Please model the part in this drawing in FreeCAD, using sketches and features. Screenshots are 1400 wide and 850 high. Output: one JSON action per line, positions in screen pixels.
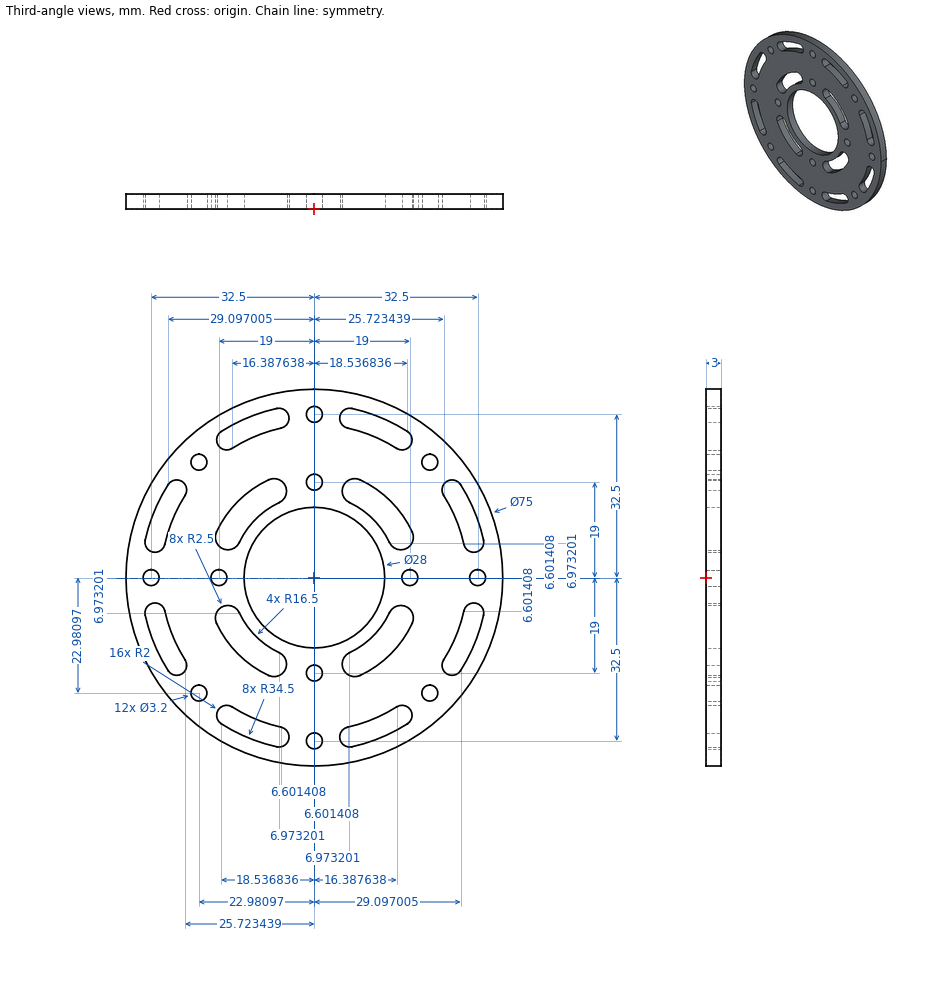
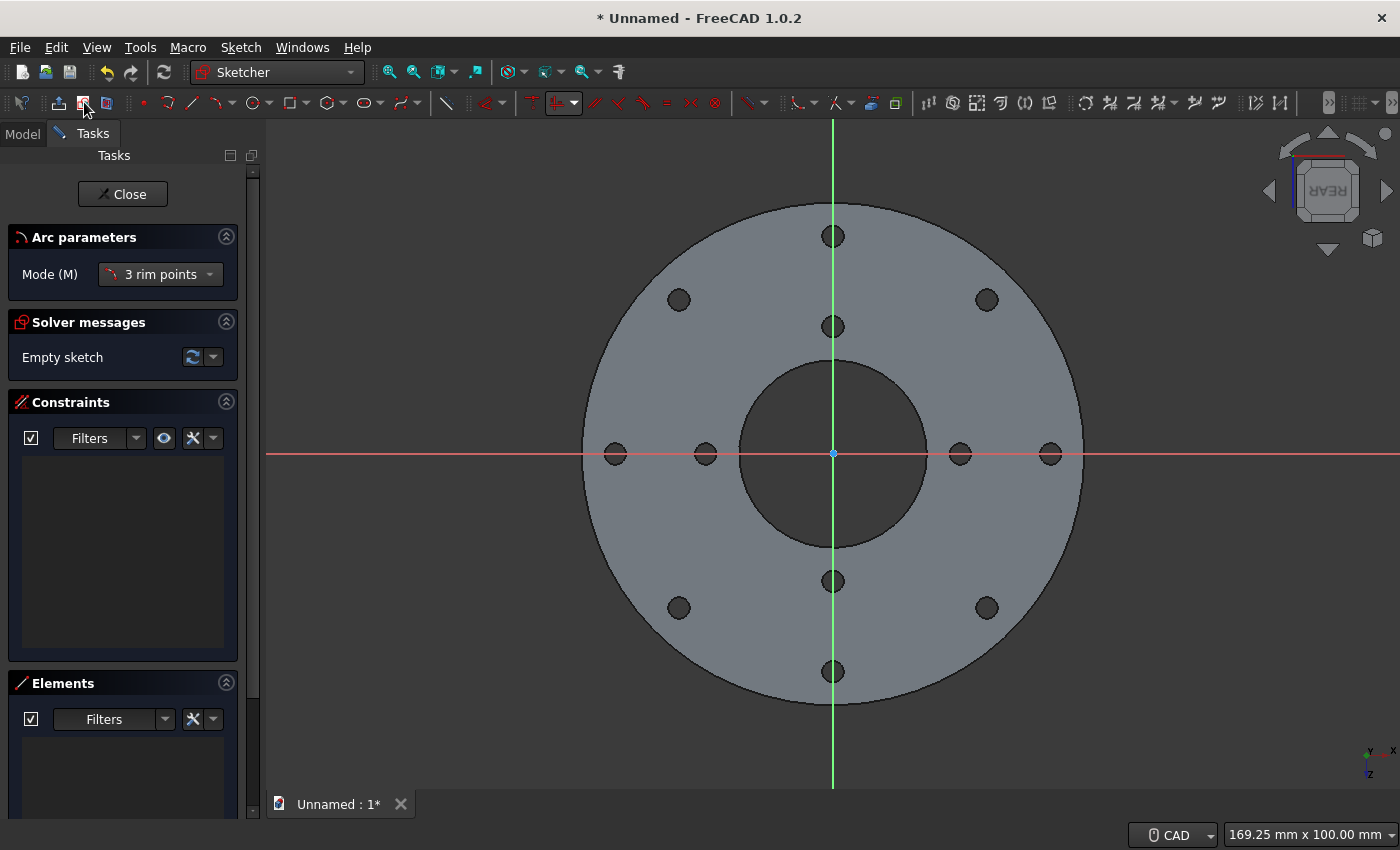
{"action": "left_click", "coordinate": [789, 254]}
{"action": "left_click", "coordinate": [783, 228]}
{"action": "left_click", "coordinate": [799, 239]}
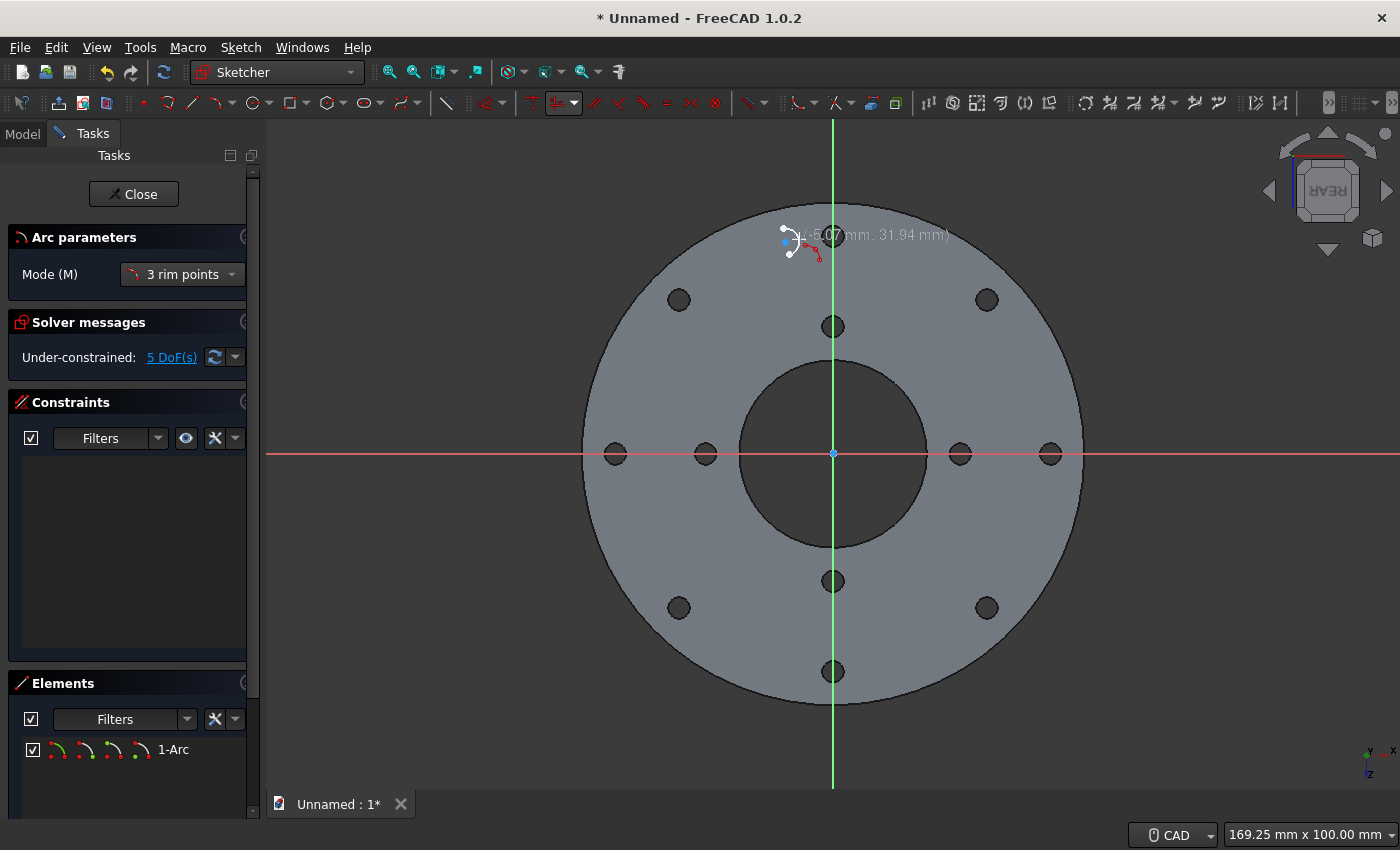
{"action": "left_click", "coordinate": [783, 229]}
{"action": "left_click", "coordinate": [709, 259]}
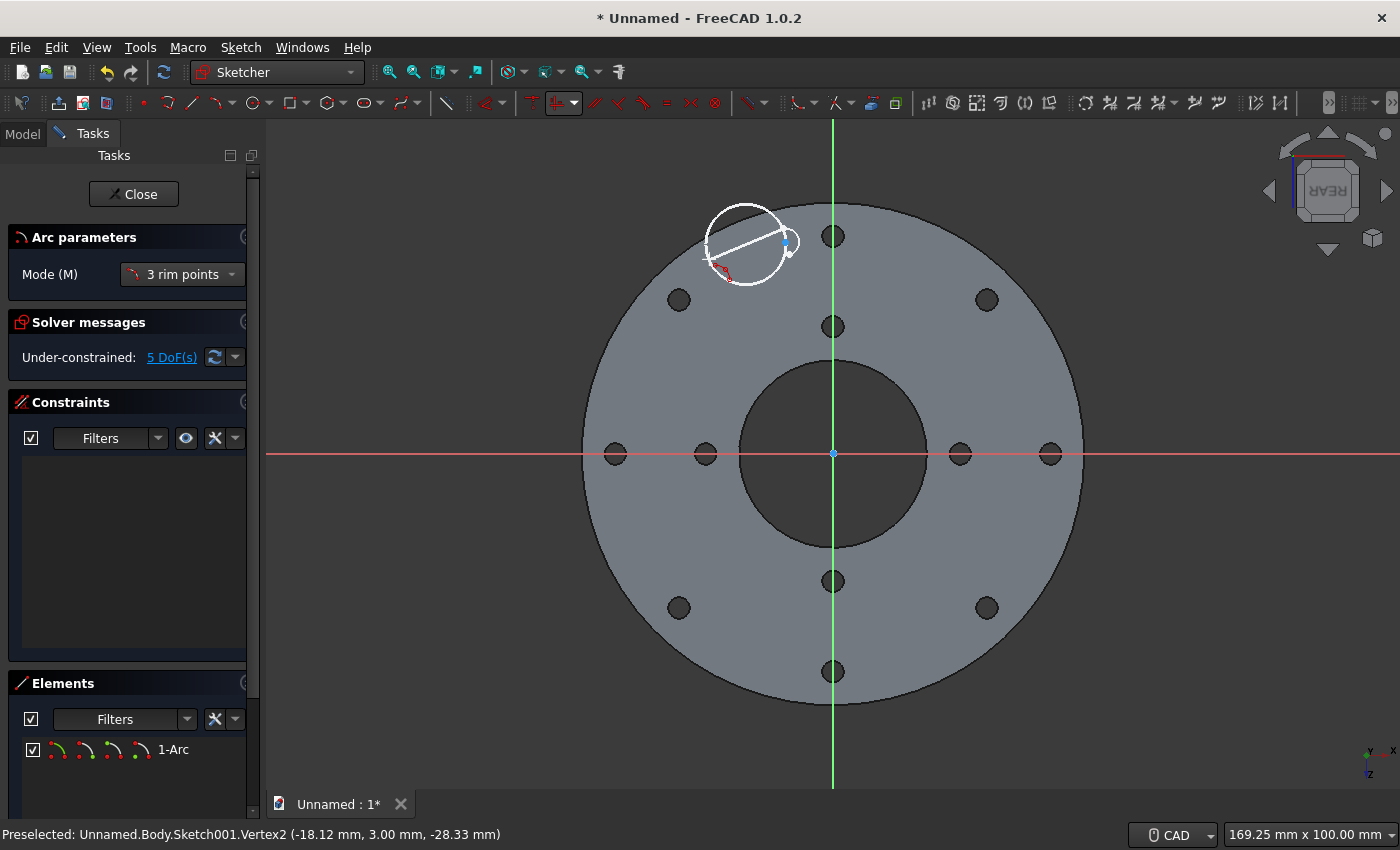
{"action": "scroll", "coordinate": [745, 240], "scroll_direction": "up", "scroll_amount": 8}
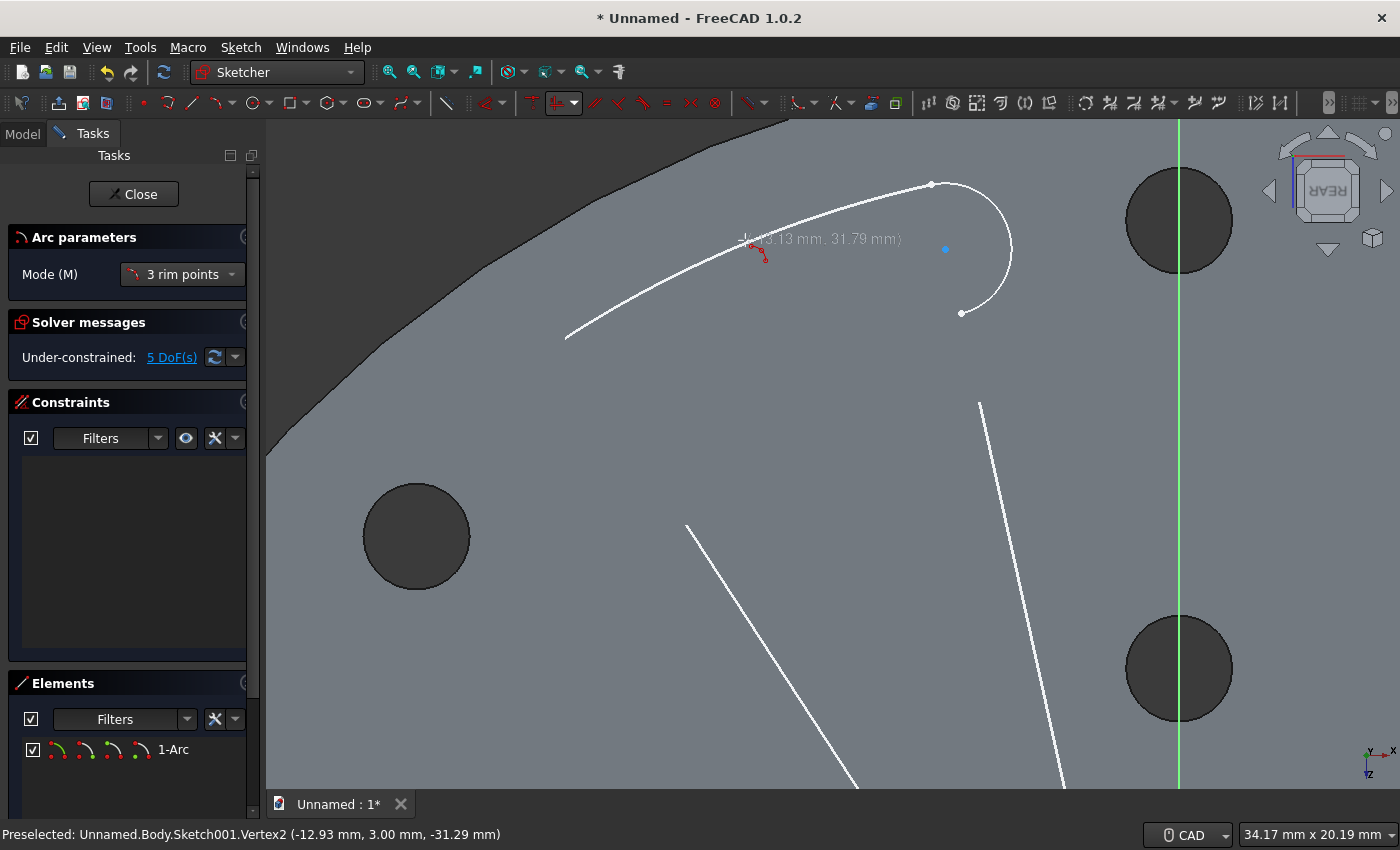
{"action": "left_click", "coordinate": [741, 241]}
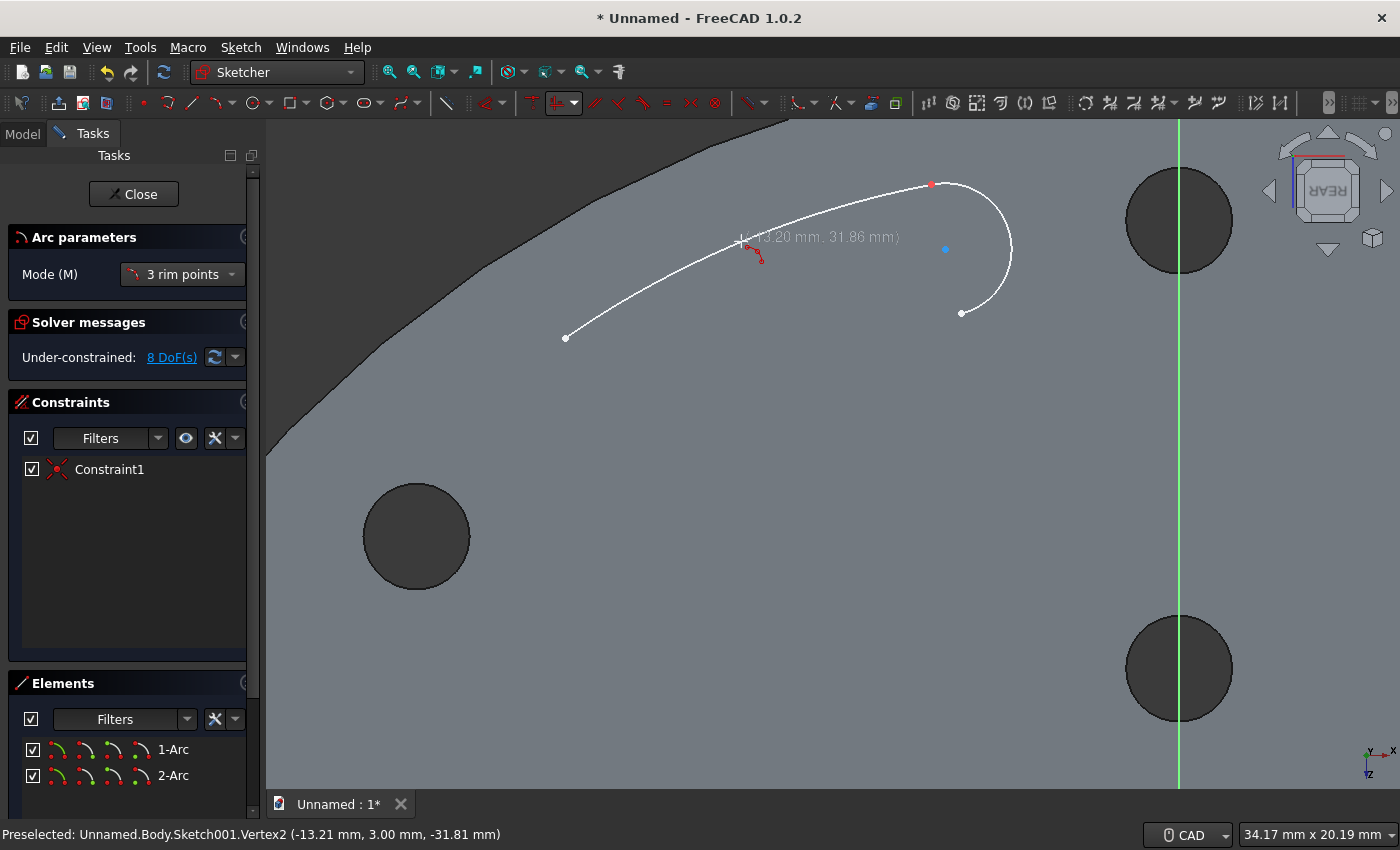
{"action": "scroll", "coordinate": [660, 240], "scroll_direction": "down", "scroll_amount": 8}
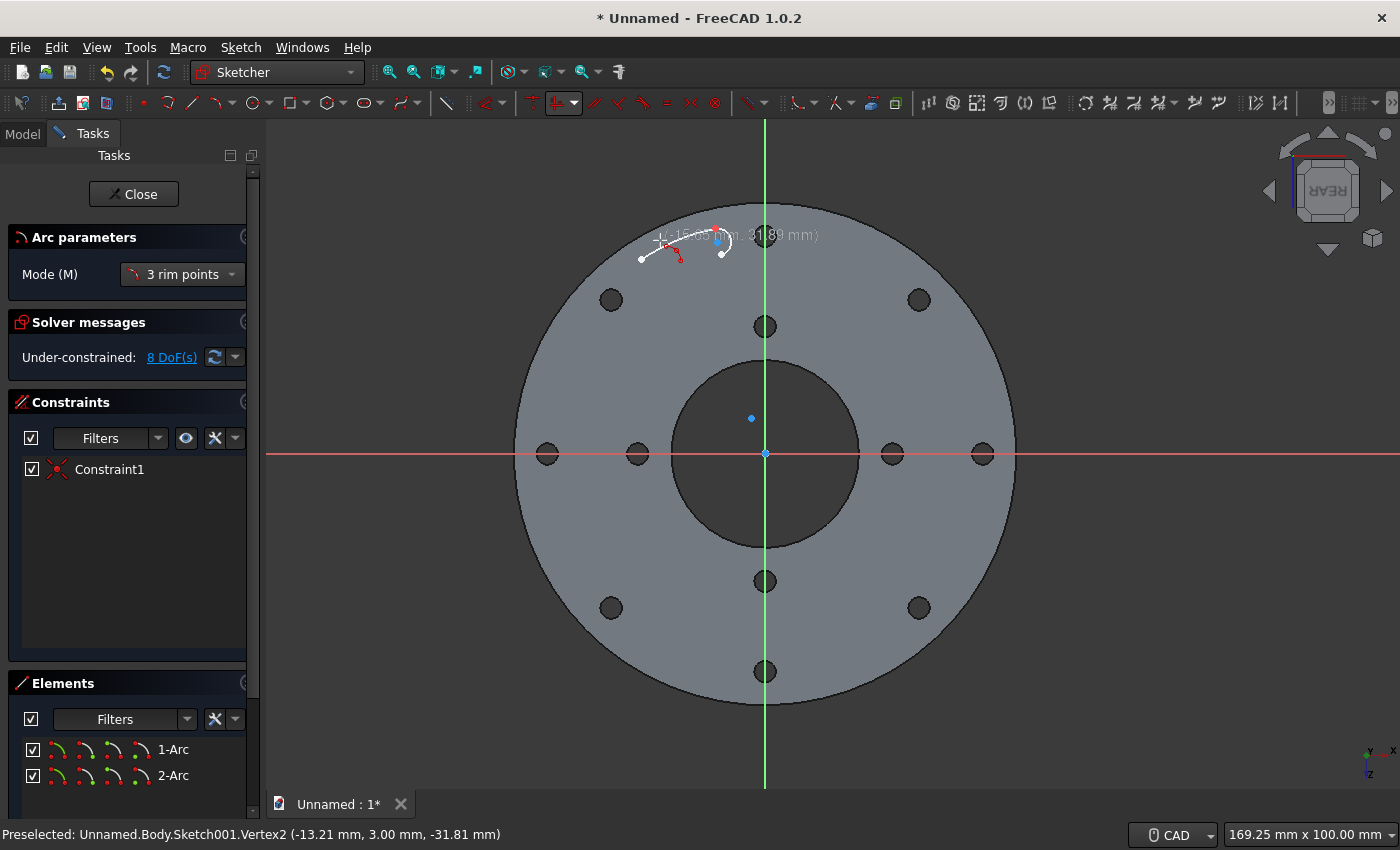
{"action": "left_click", "coordinate": [641, 260]}
{"action": "left_click", "coordinate": [655, 282]}
{"action": "left_click", "coordinate": [637, 278]}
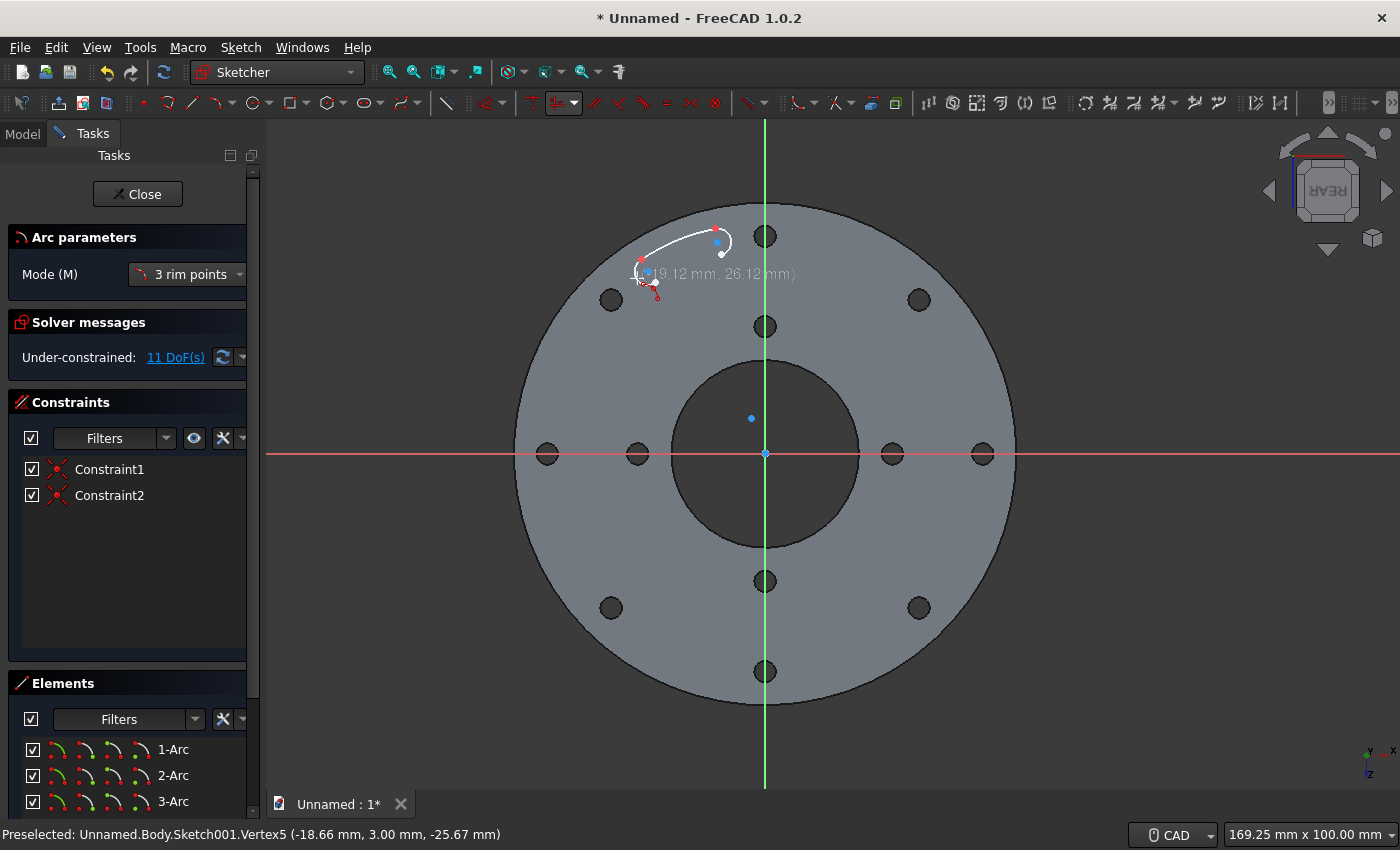
{"action": "left_click", "coordinate": [655, 283]}
{"action": "left_click", "coordinate": [721, 255]}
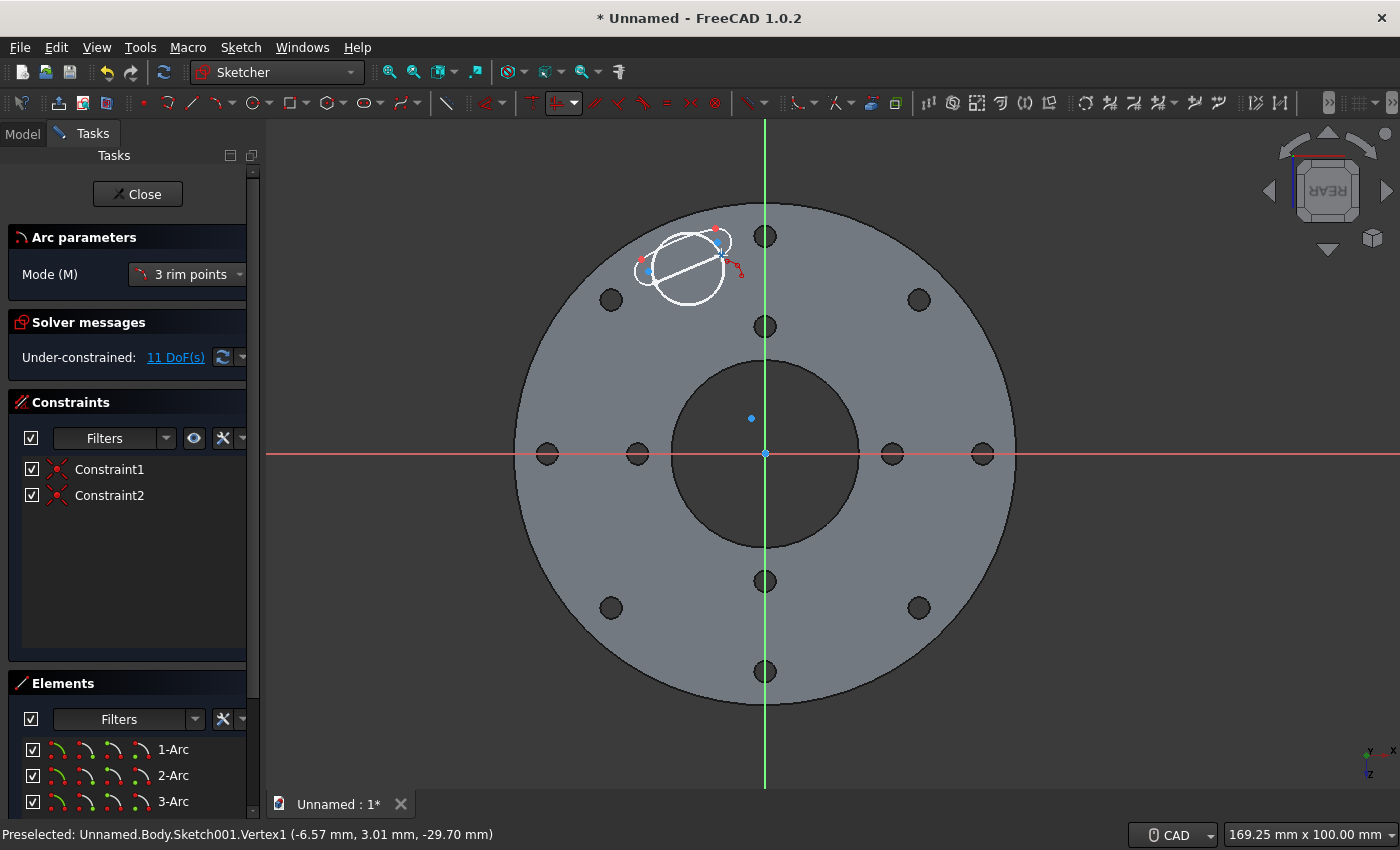
{"action": "scroll", "coordinate": [687, 265], "scroll_direction": "up", "scroll_amount": 9}